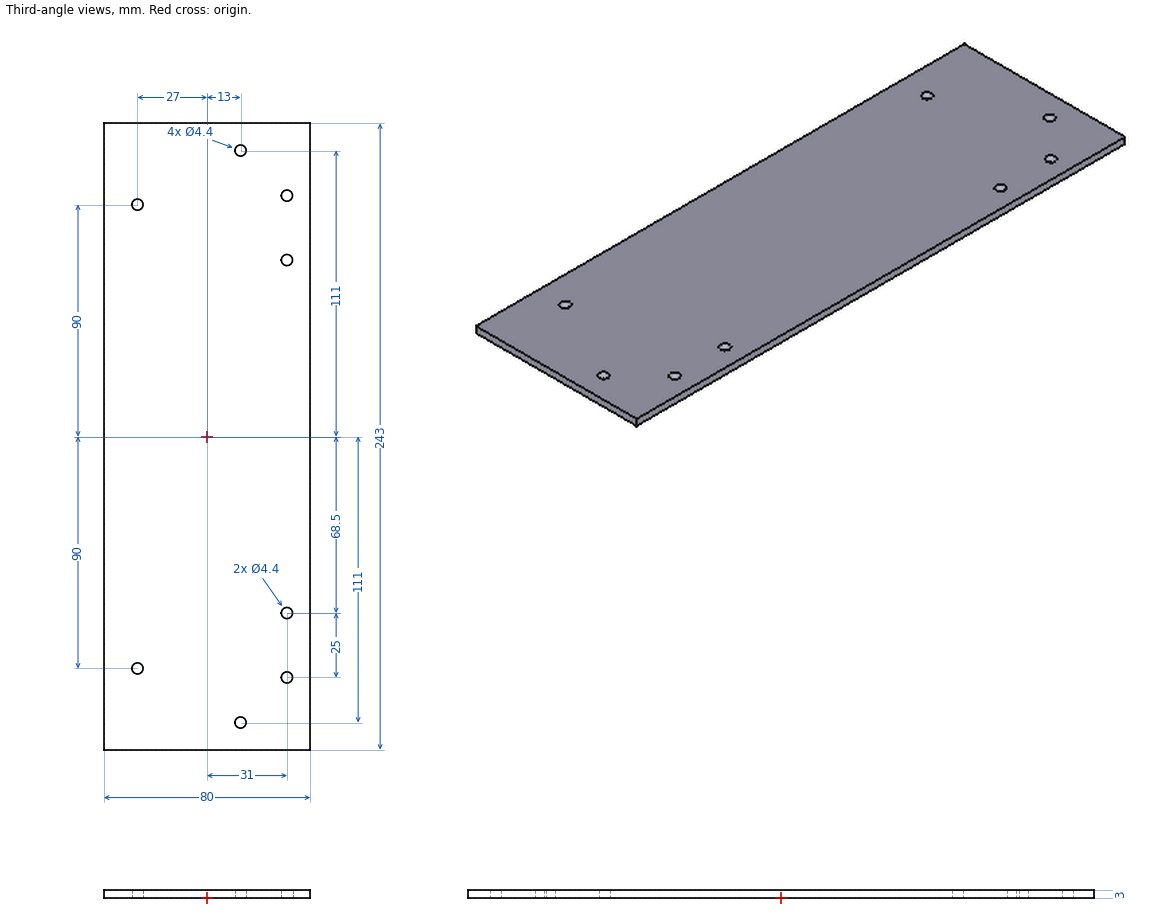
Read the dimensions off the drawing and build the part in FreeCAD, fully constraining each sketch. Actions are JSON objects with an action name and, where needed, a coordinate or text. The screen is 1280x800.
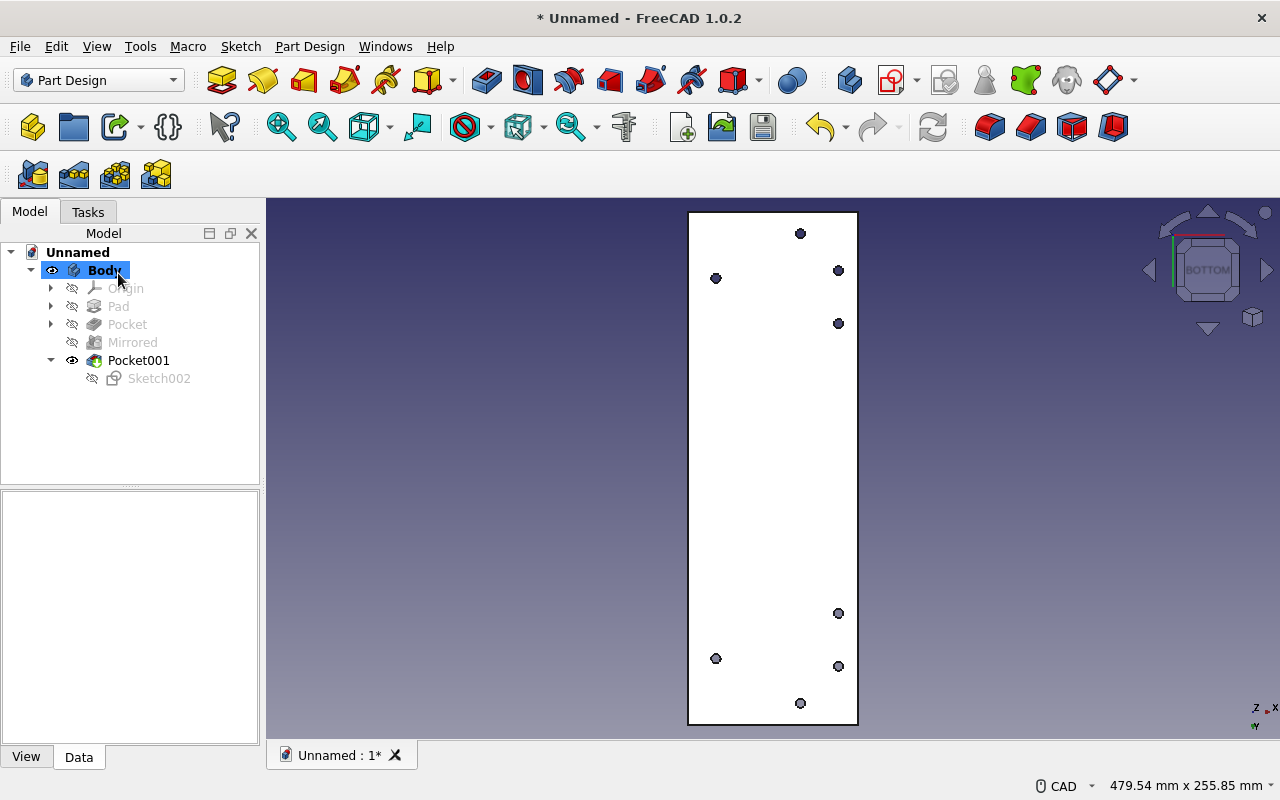
{"action": "key", "text": "0"}